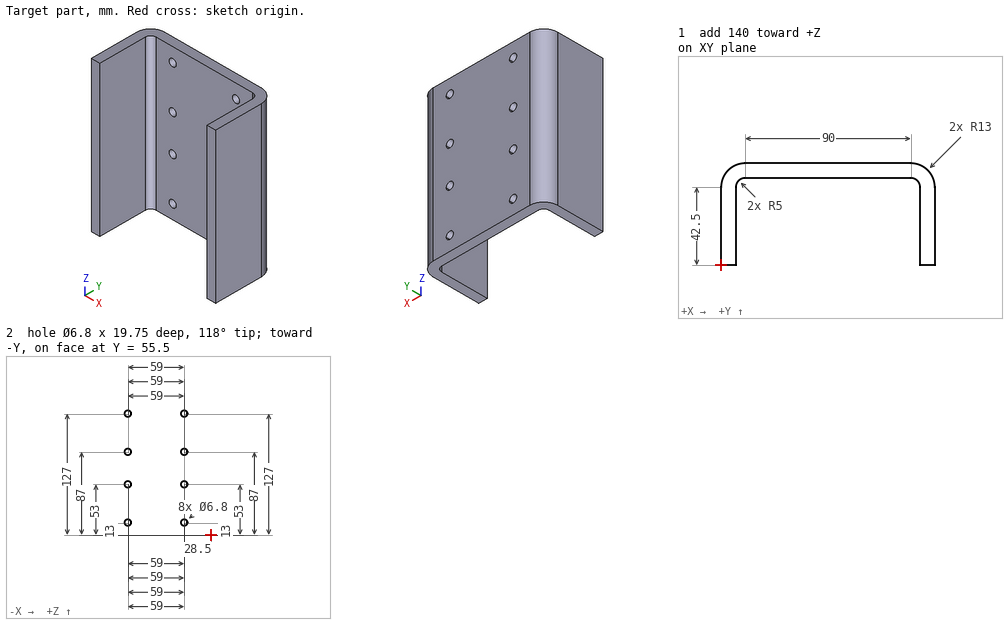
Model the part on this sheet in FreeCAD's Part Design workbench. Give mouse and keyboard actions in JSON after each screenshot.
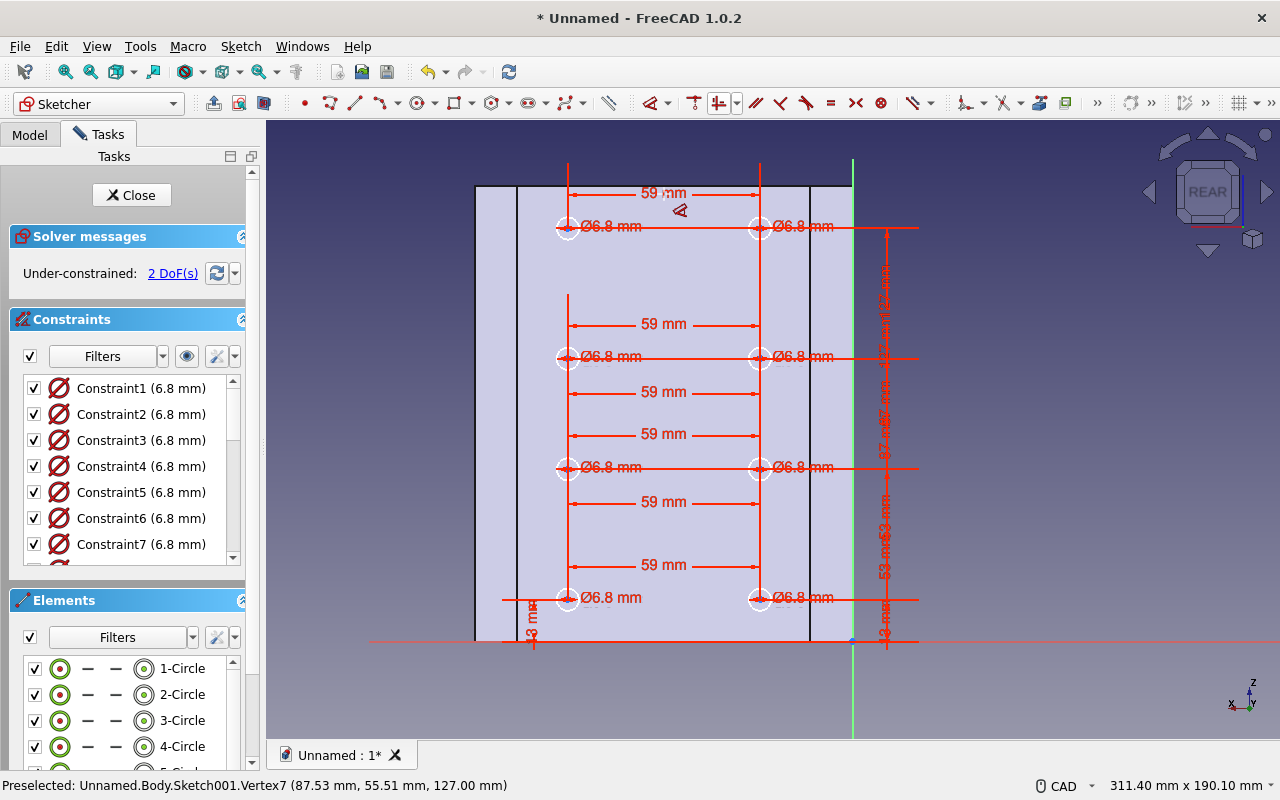
{"action": "left_click", "coordinate": [568, 228]}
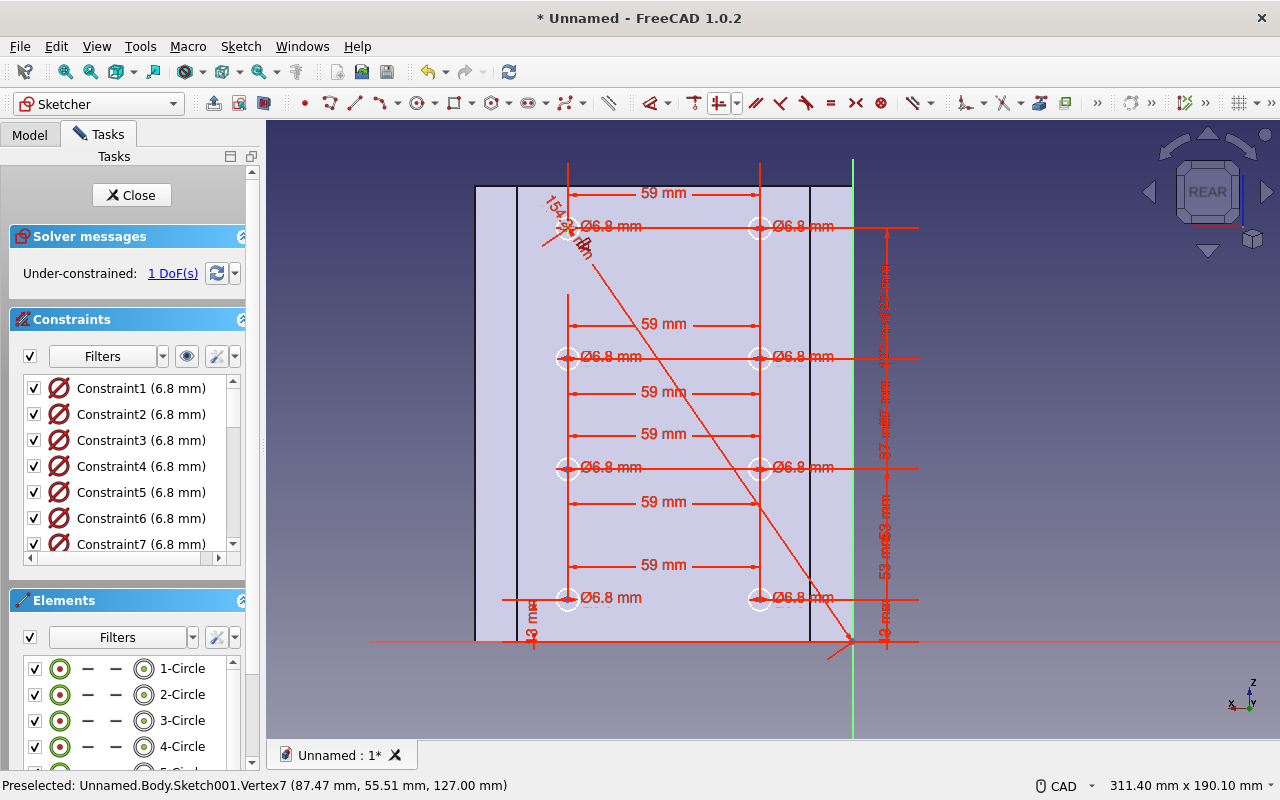
{"action": "left_click", "coordinate": [760, 228]}
{"action": "left_click", "coordinate": [664, 262]}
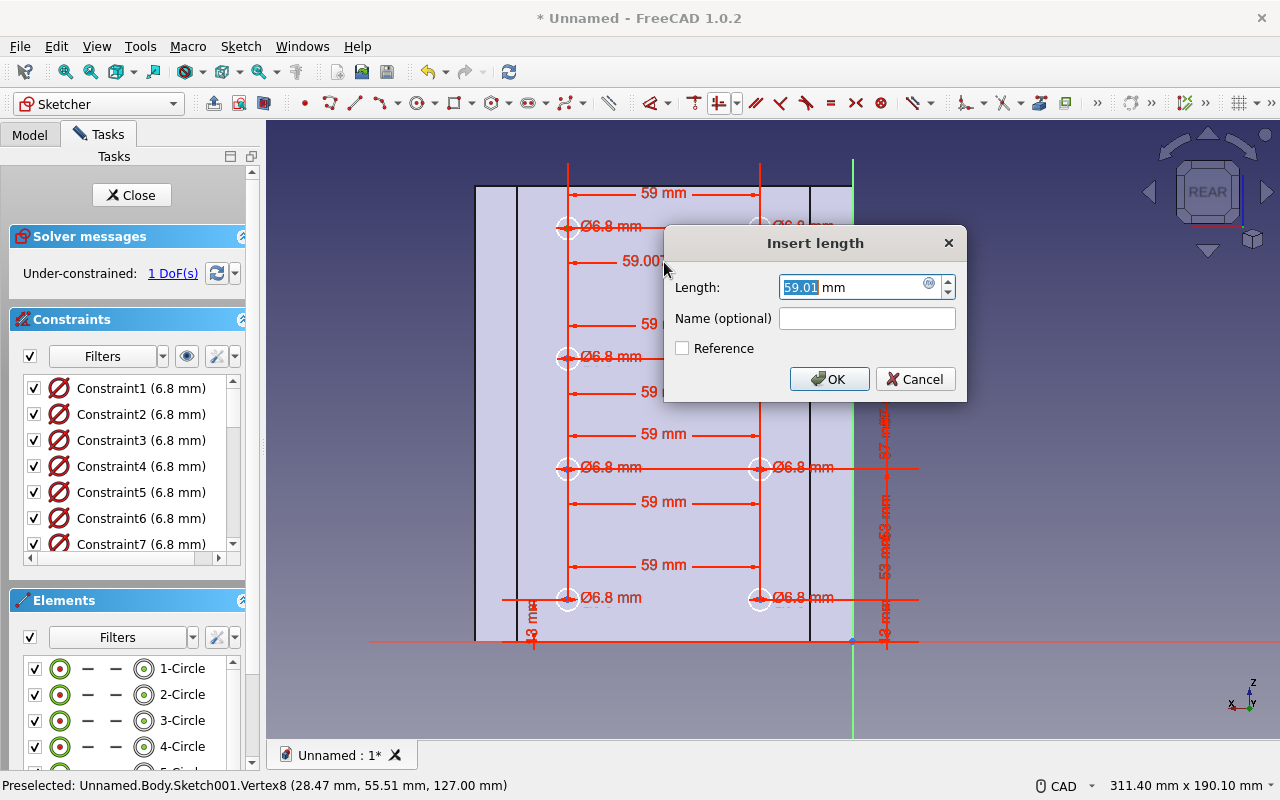
{"action": "type", "text": "59"}
{"action": "key", "text": "Return"}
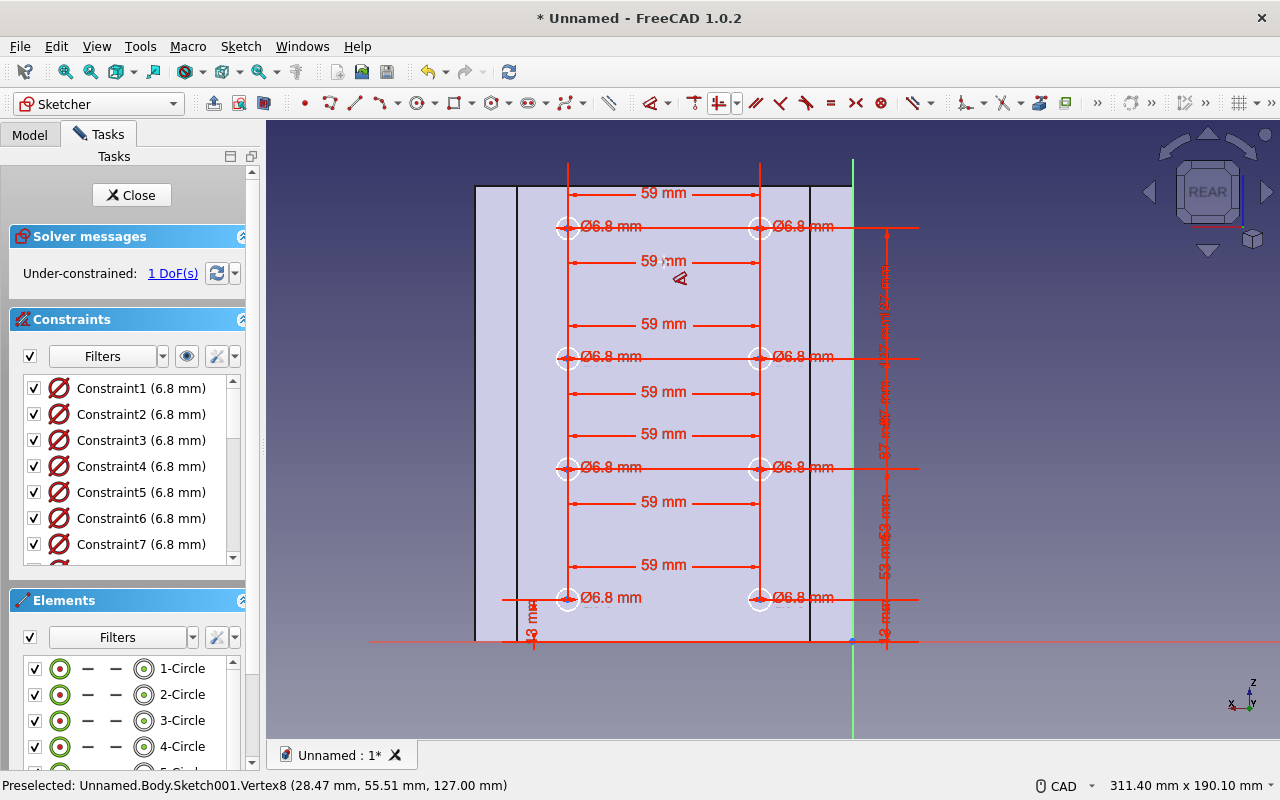
{"action": "left_click", "coordinate": [760, 600]}
{"action": "left_click", "coordinate": [806, 676]}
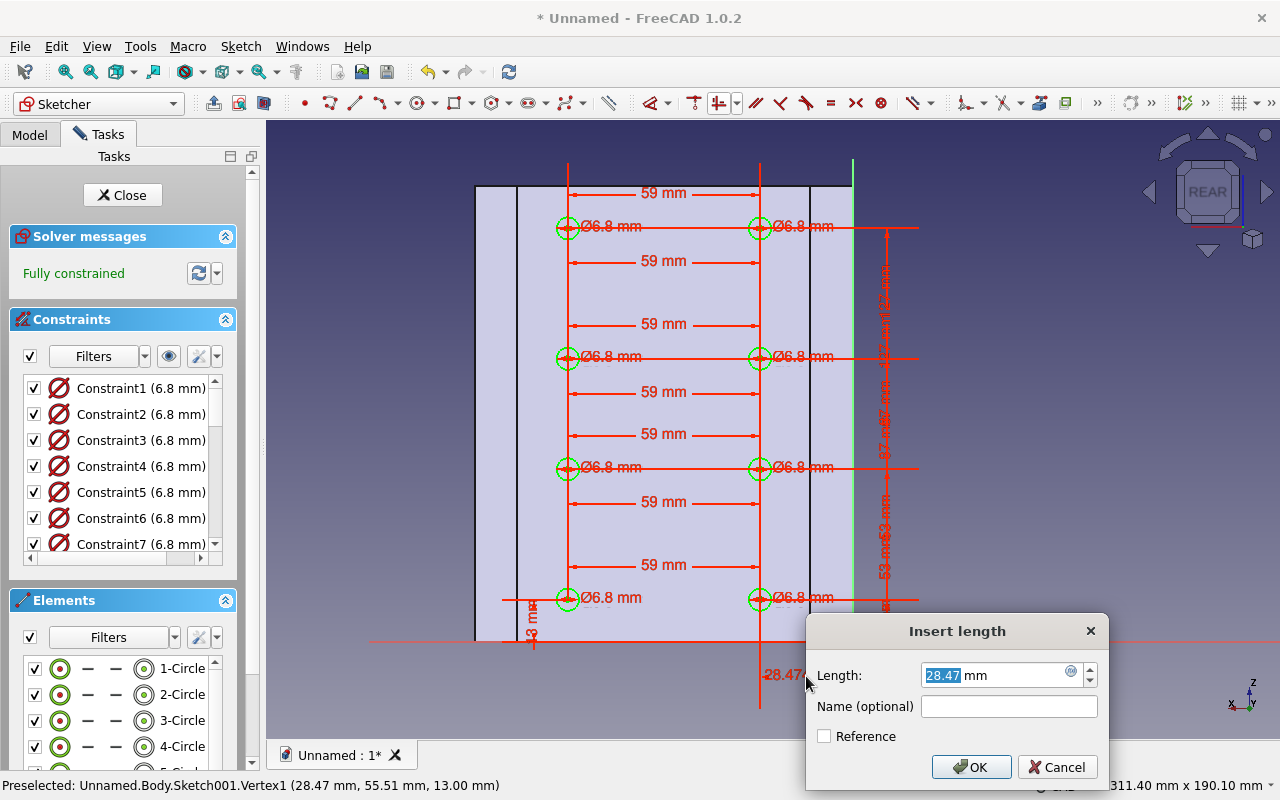
{"action": "type", "text": "28.5"}
{"action": "key", "text": "Return"}
{"action": "key", "text": "Escape"}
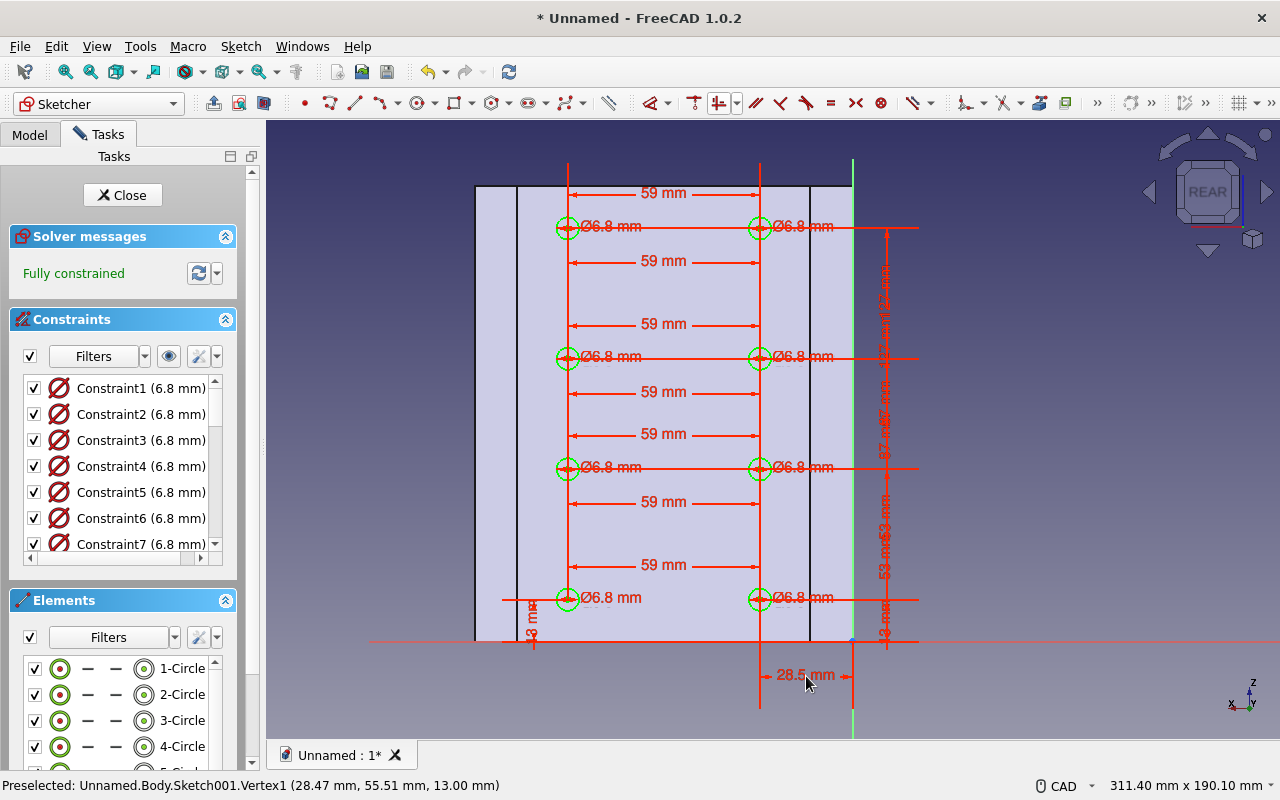
{"action": "left_click", "coordinate": [123, 195]}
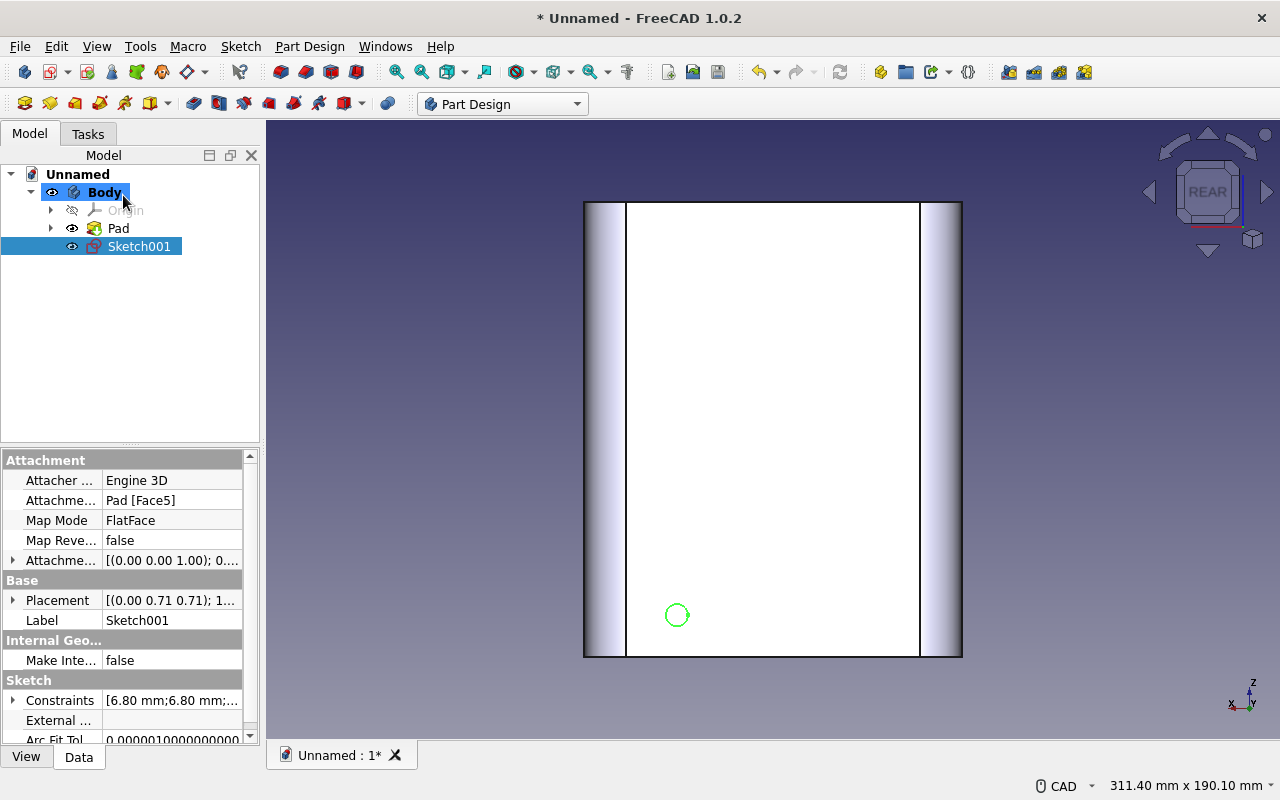
{"action": "left_click", "coordinate": [219, 104]}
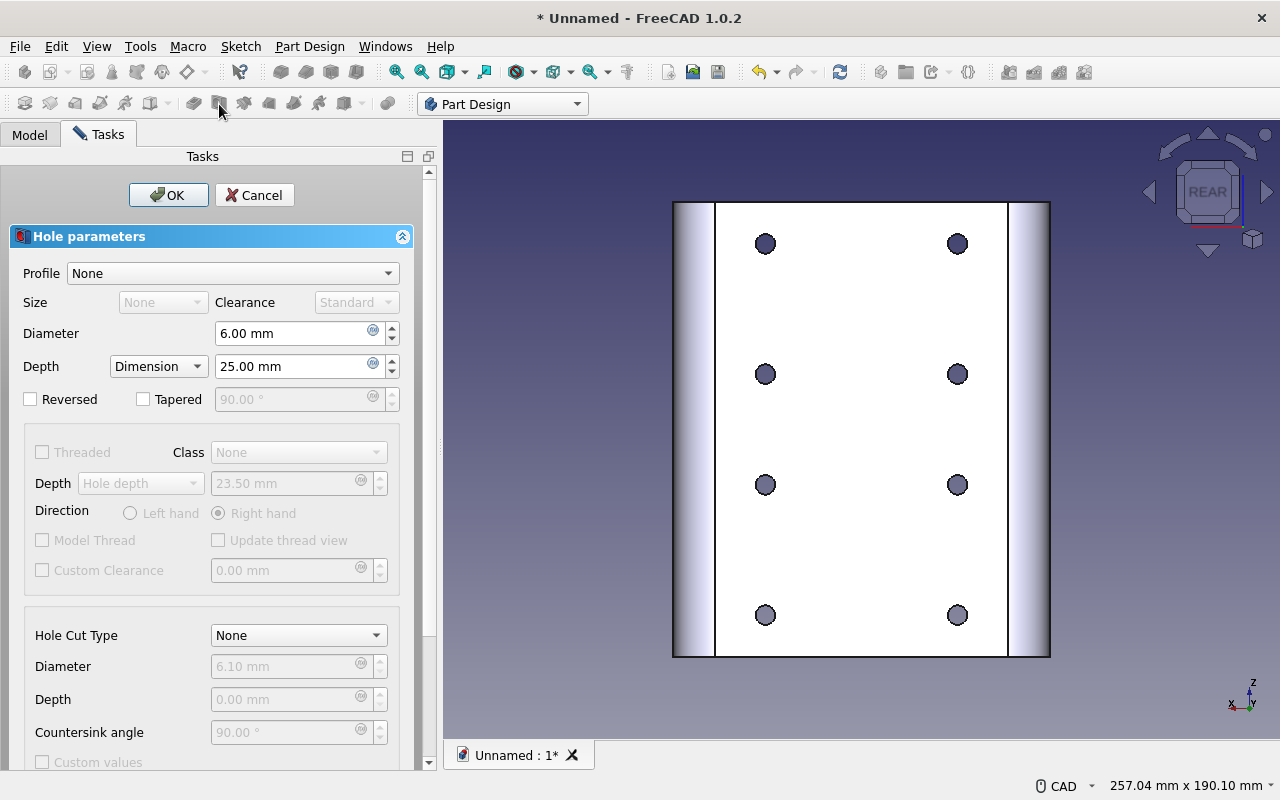
{"action": "triple_click", "coordinate": [300, 334]}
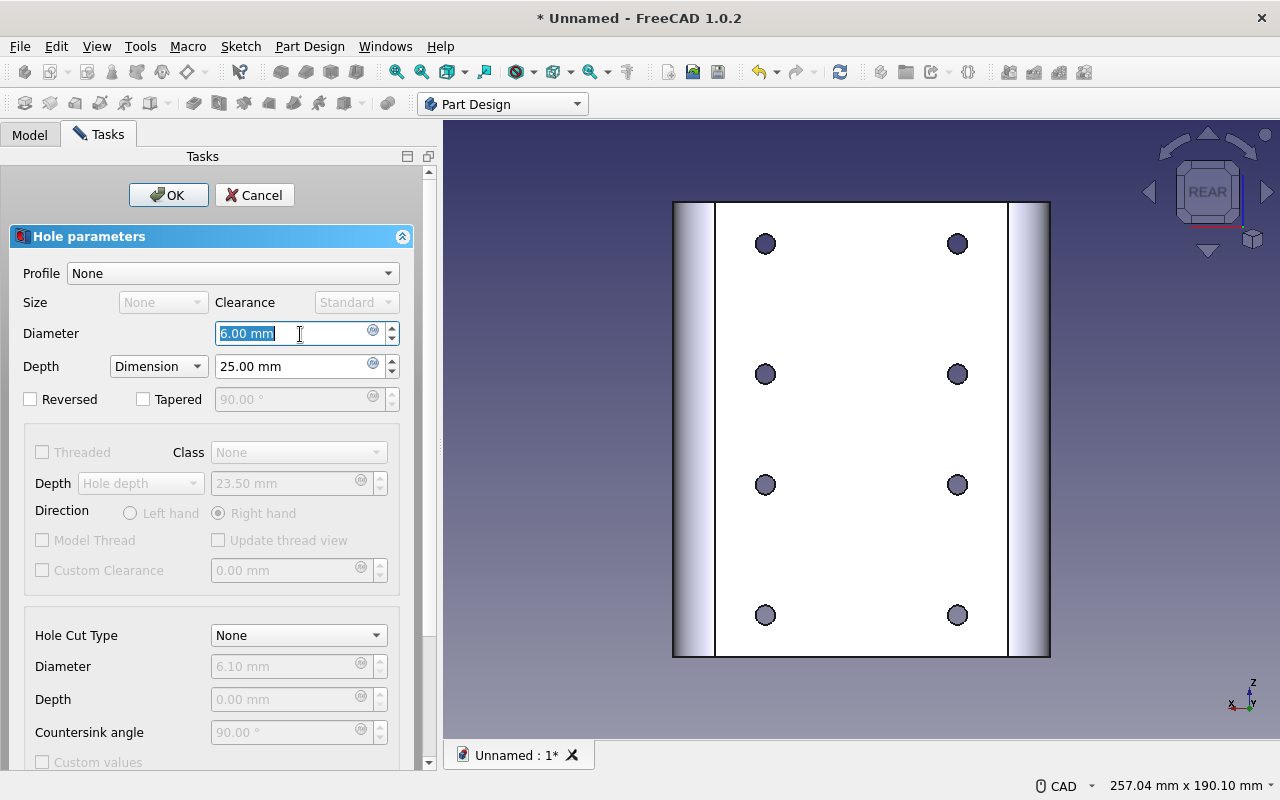
{"action": "type", "text": "6.8"}
{"action": "key", "text": "Tab"}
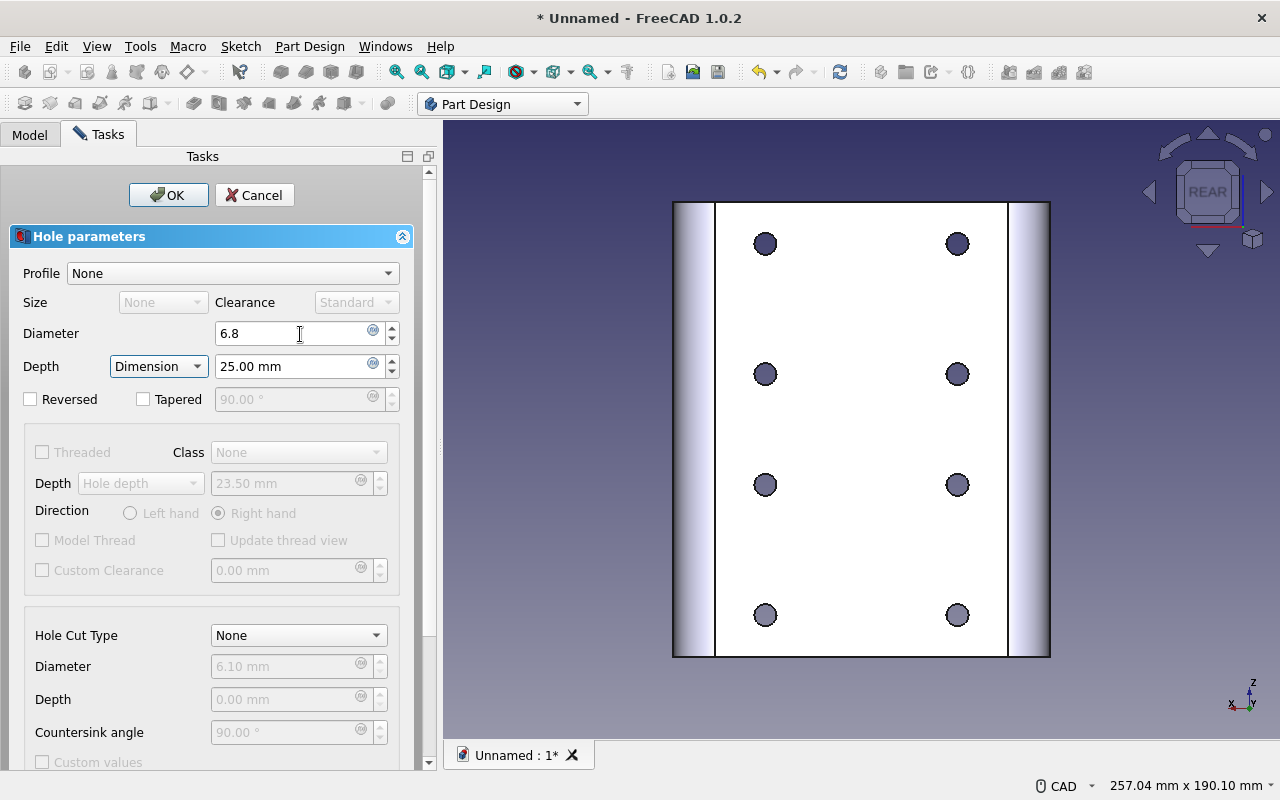
{"action": "triple_click", "coordinate": [300, 366]}